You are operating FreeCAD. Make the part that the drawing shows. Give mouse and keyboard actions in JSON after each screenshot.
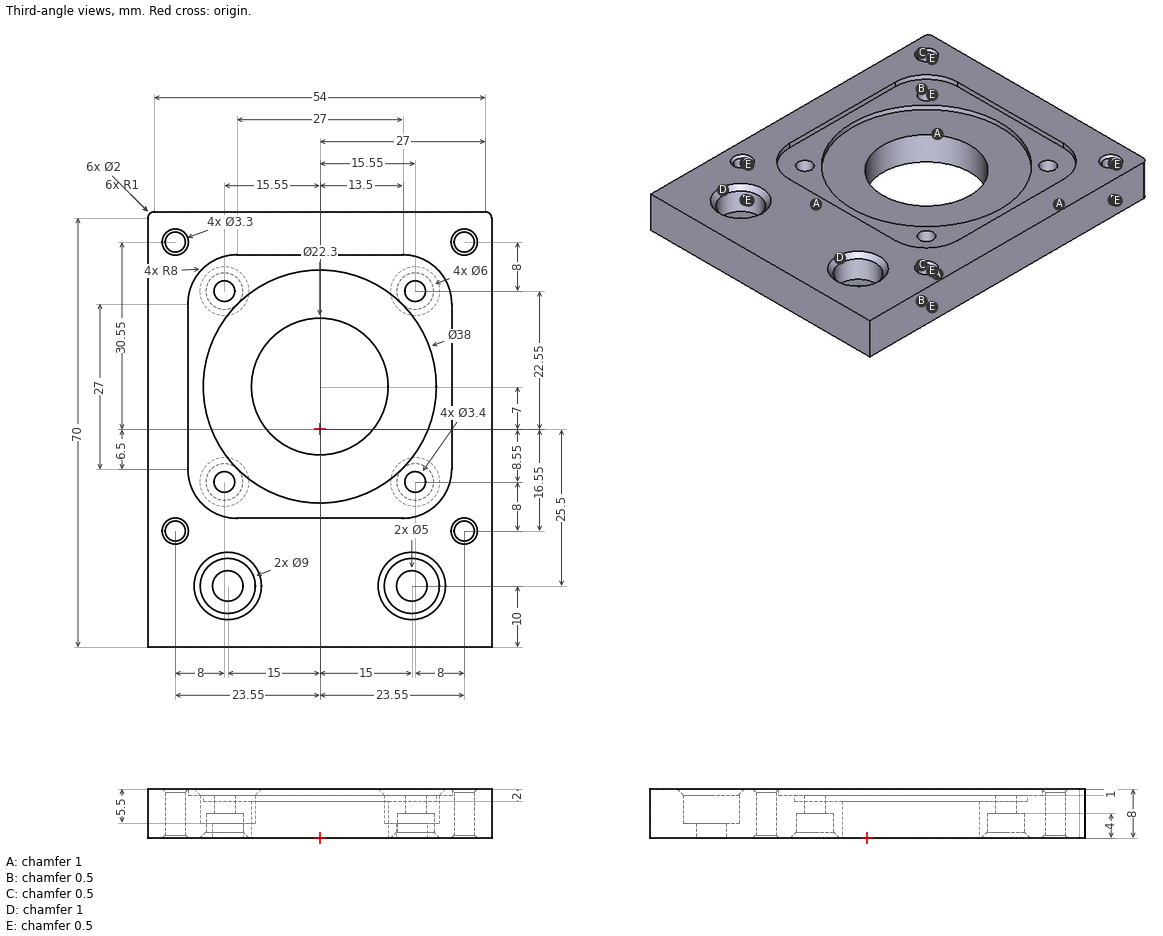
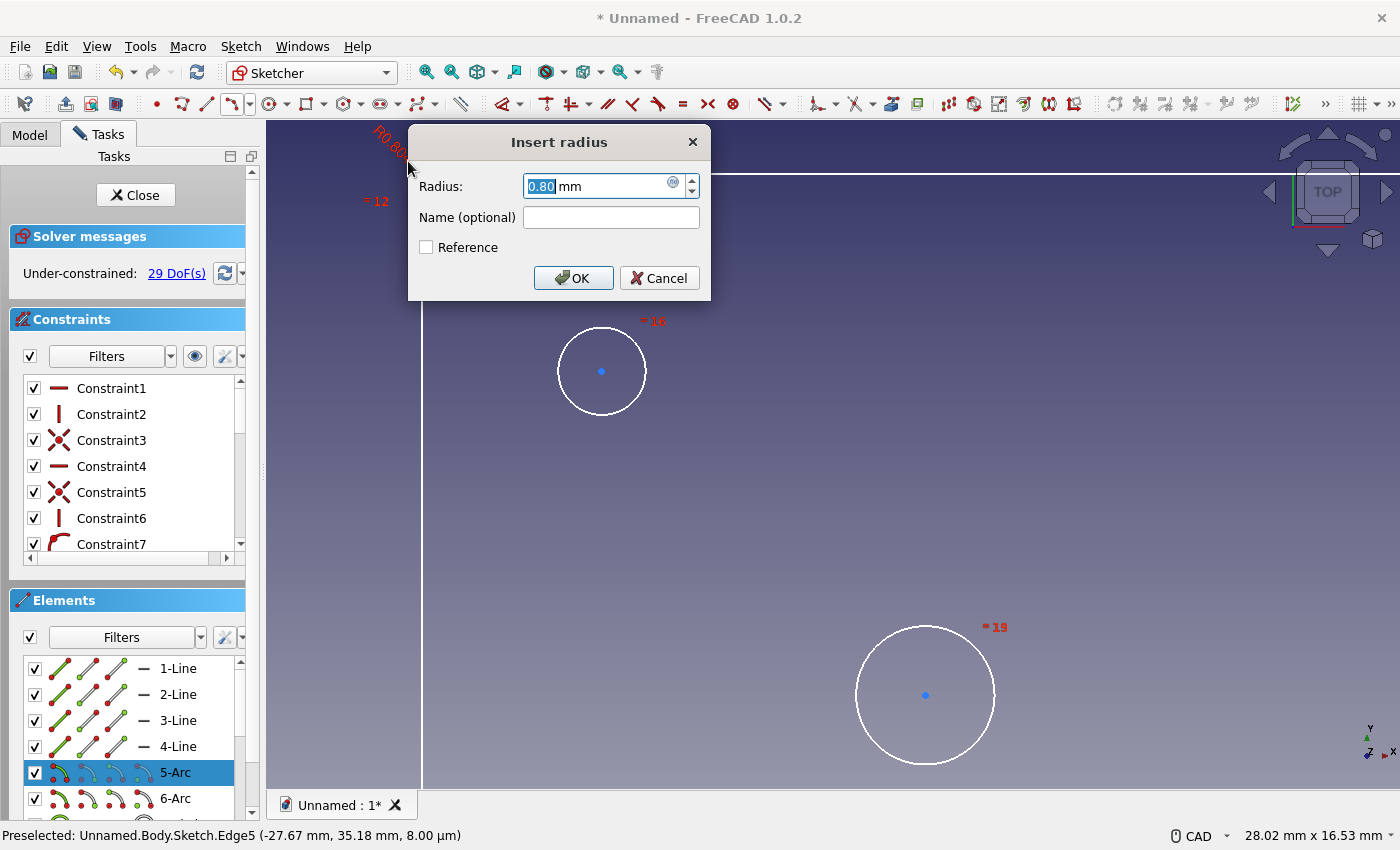
{"action": "type", "text": "1"}
{"action": "key", "text": "Return"}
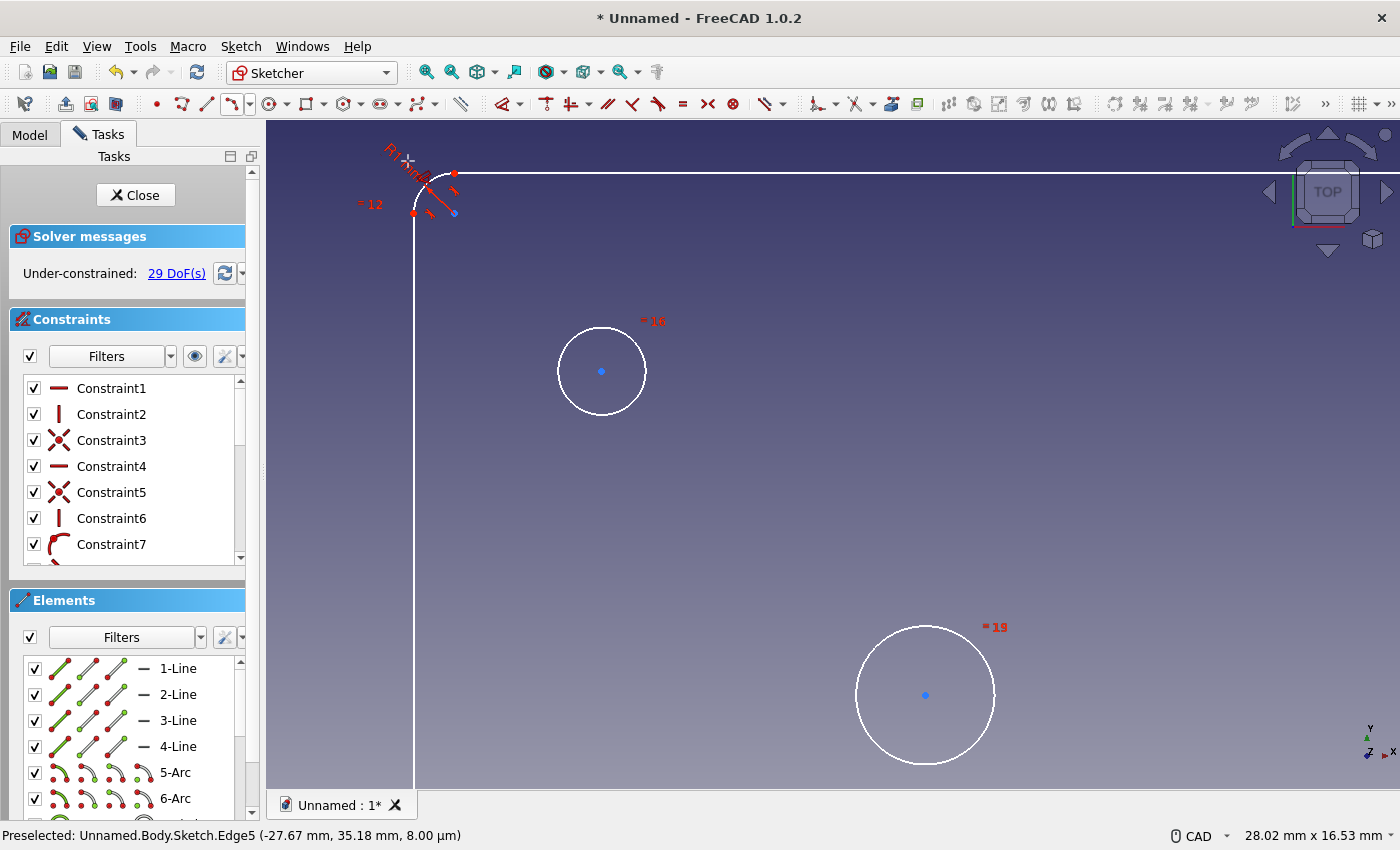
{"action": "scroll", "coordinate": [608, 227], "scroll_direction": "down", "scroll_amount": 9}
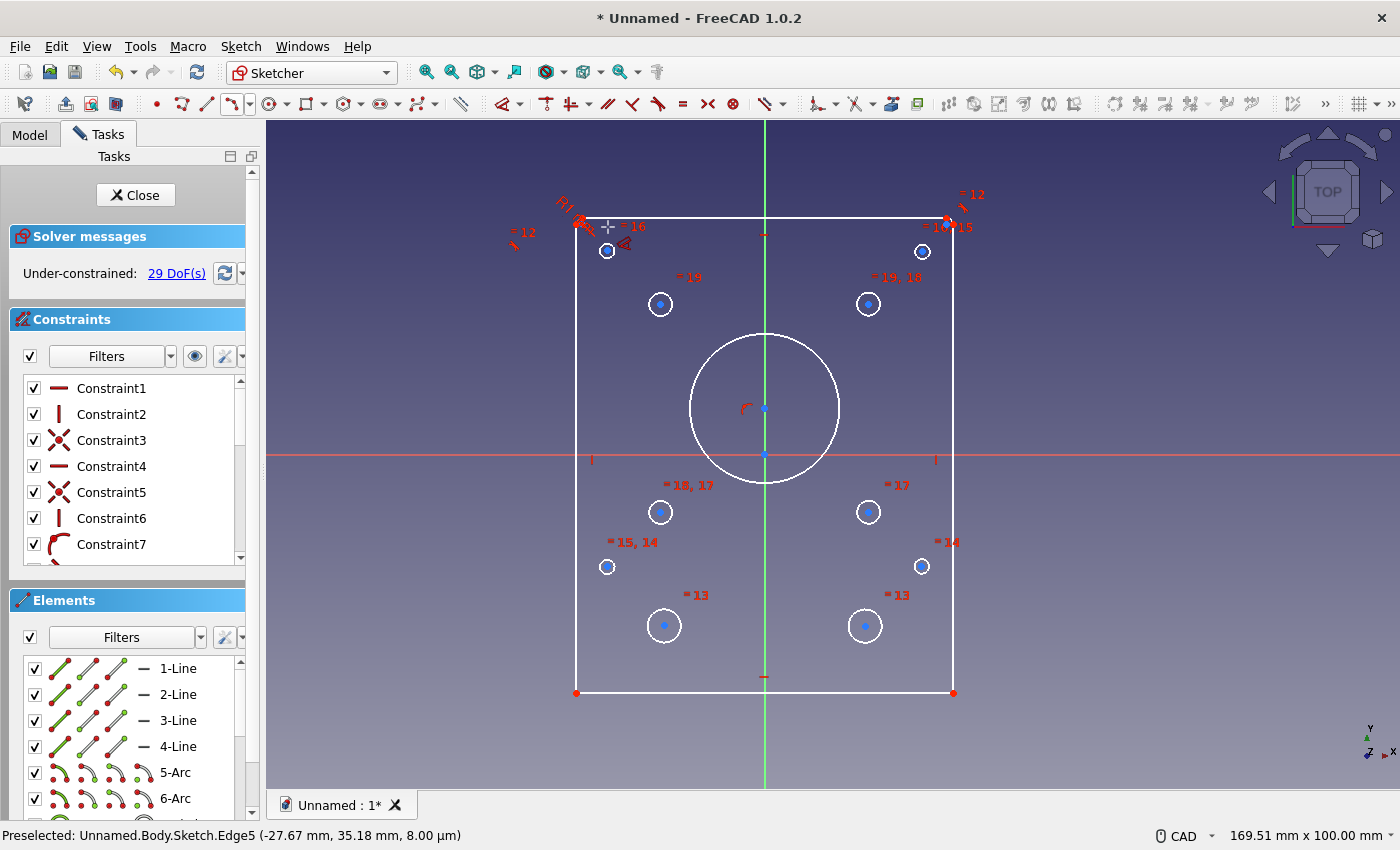
{"action": "left_click", "coordinate": [877, 614]}
{"action": "left_click", "coordinate": [899, 591]}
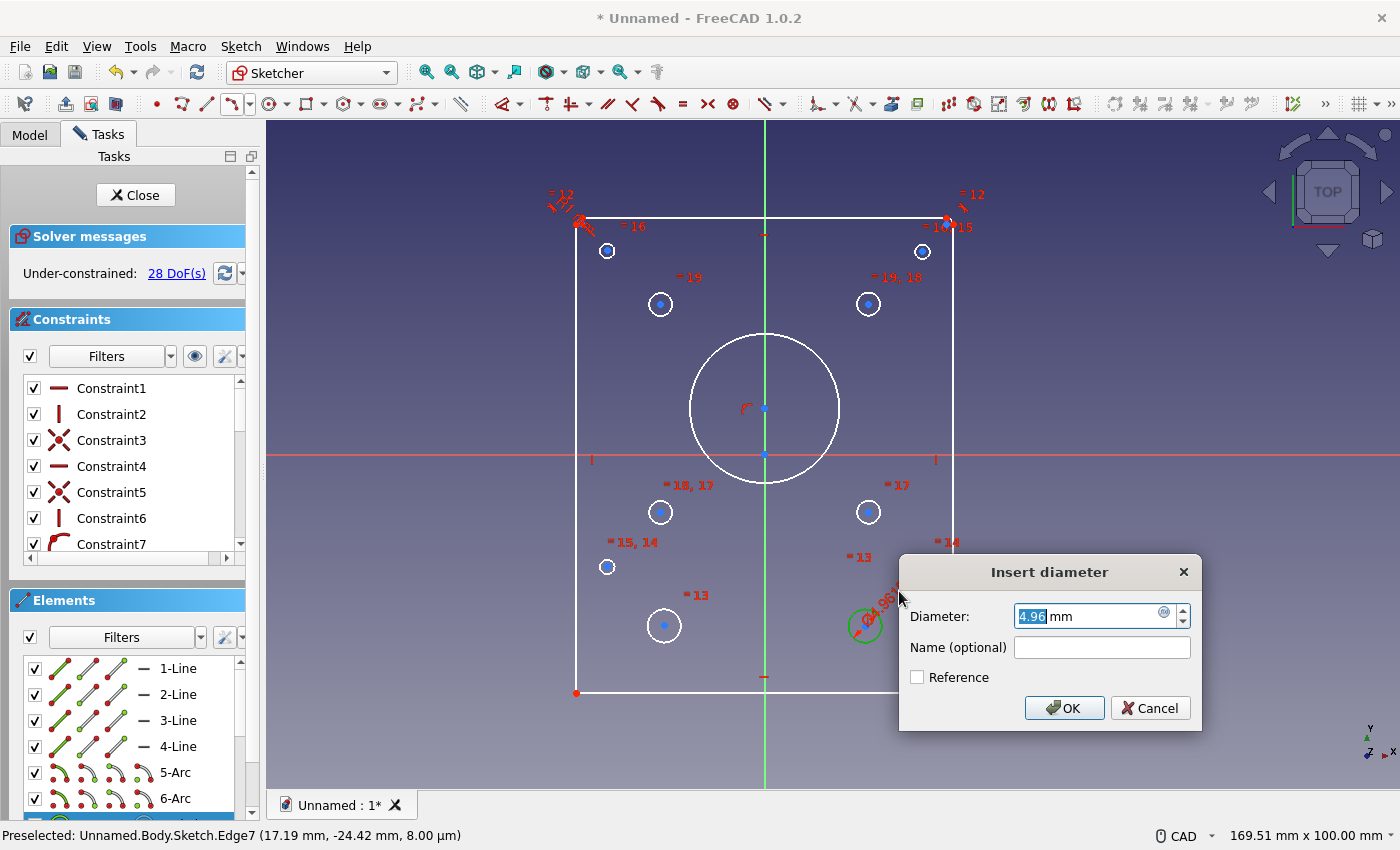
{"action": "type", "text": "5"}
{"action": "key", "text": "Return"}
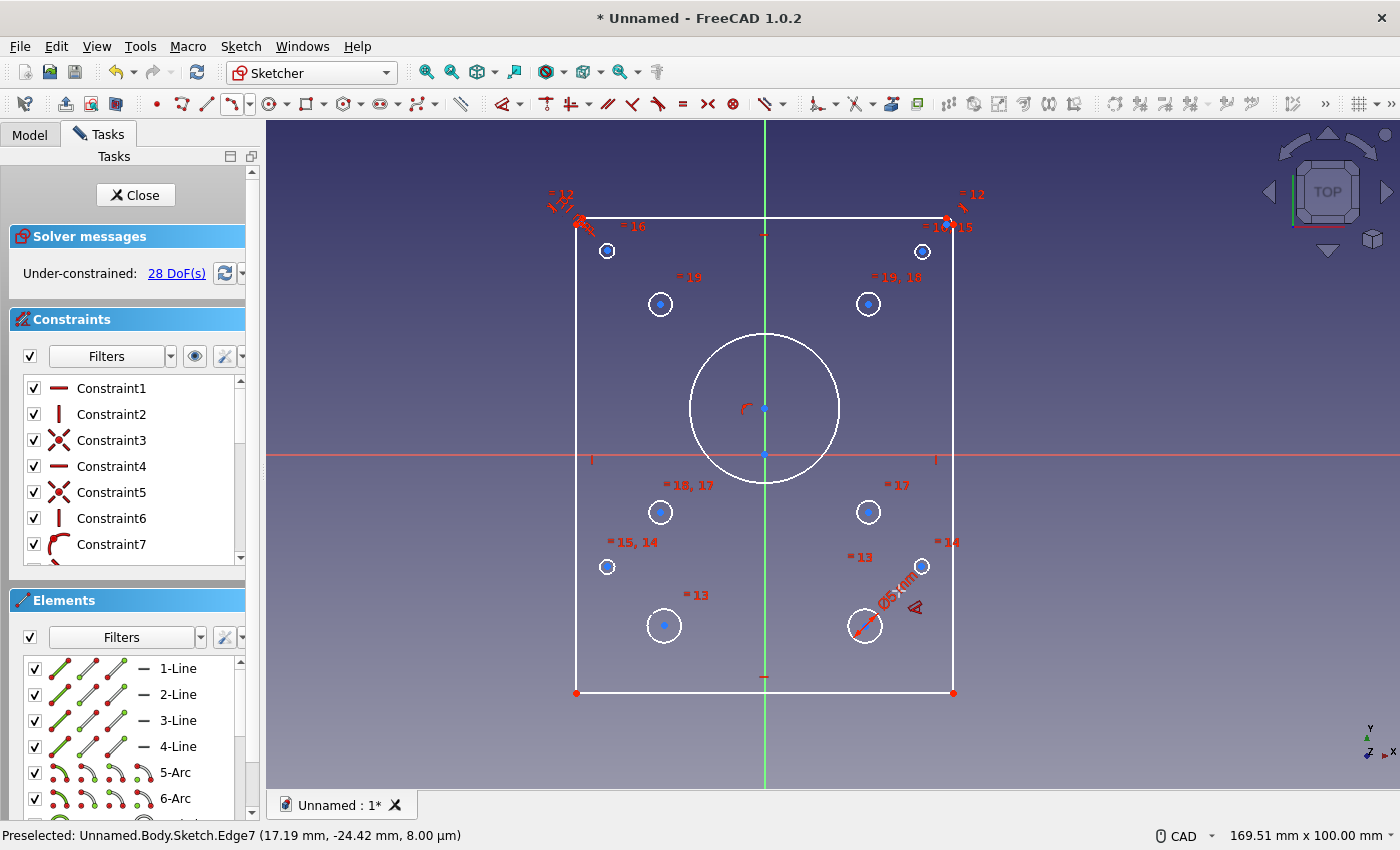
{"action": "scroll", "coordinate": [917, 561], "scroll_direction": "up", "scroll_amount": 6}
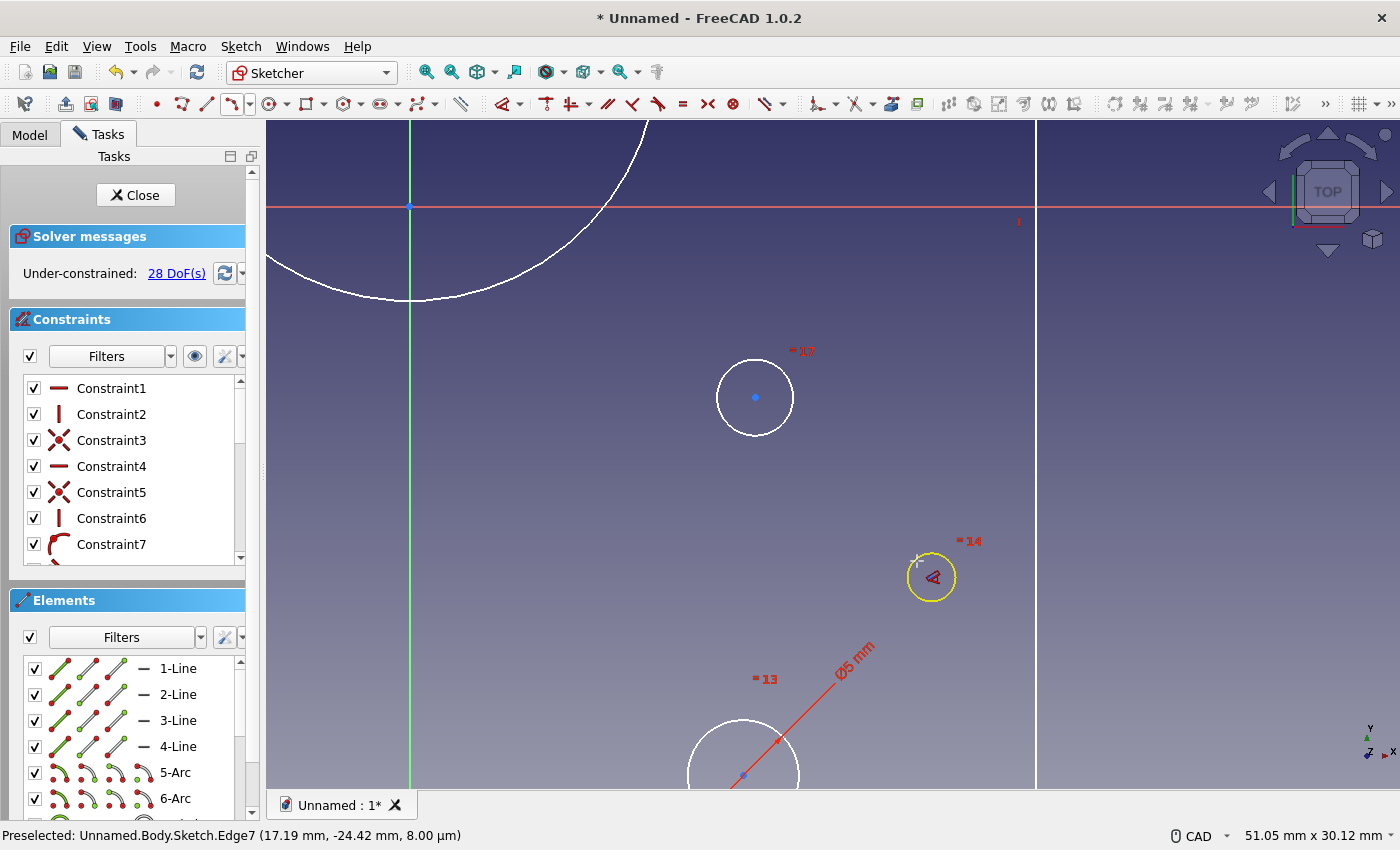
{"action": "left_click", "coordinate": [915, 560]}
{"action": "left_click", "coordinate": [893, 537]}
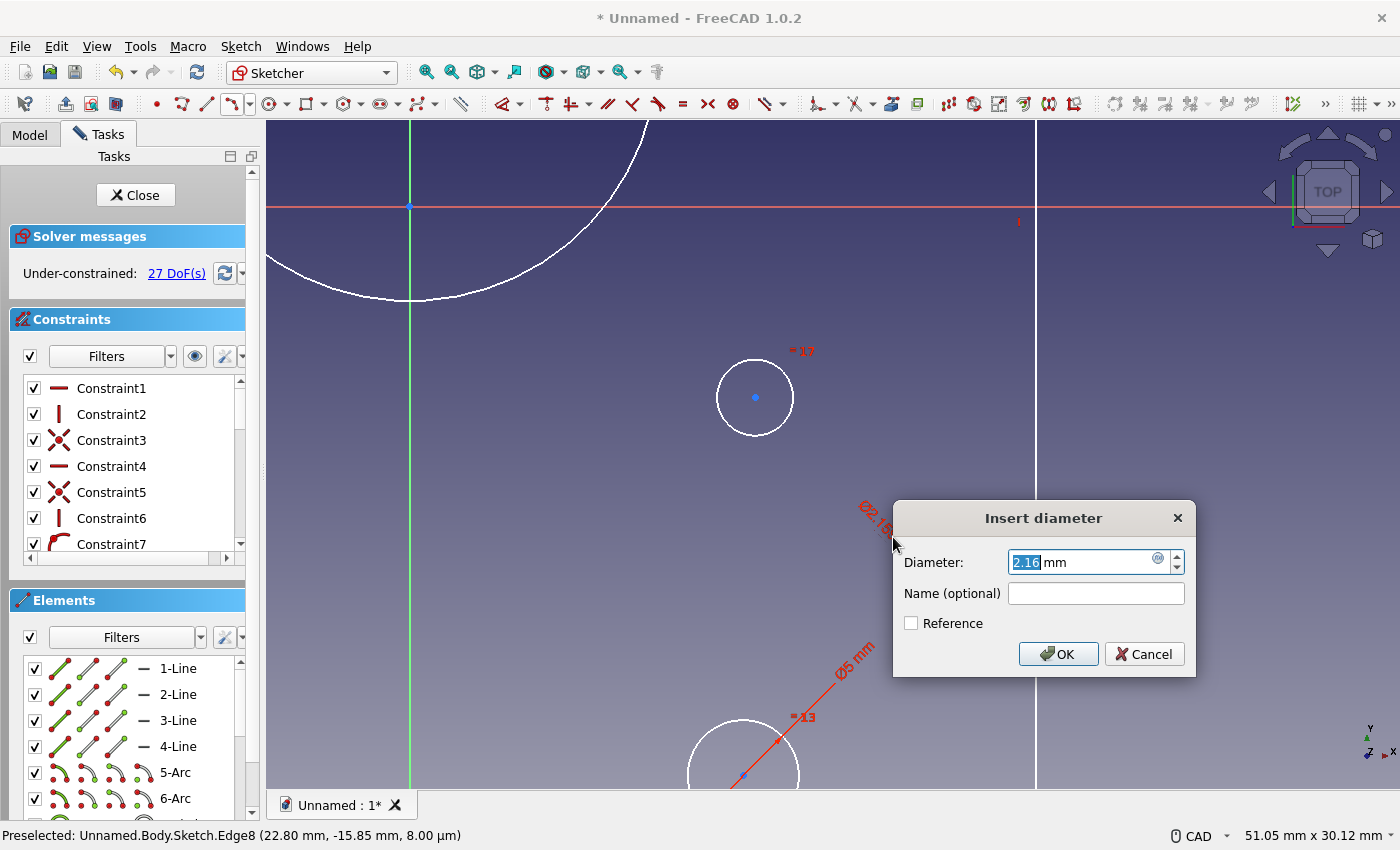
{"action": "type", "text": "2"}
{"action": "key", "text": "Return"}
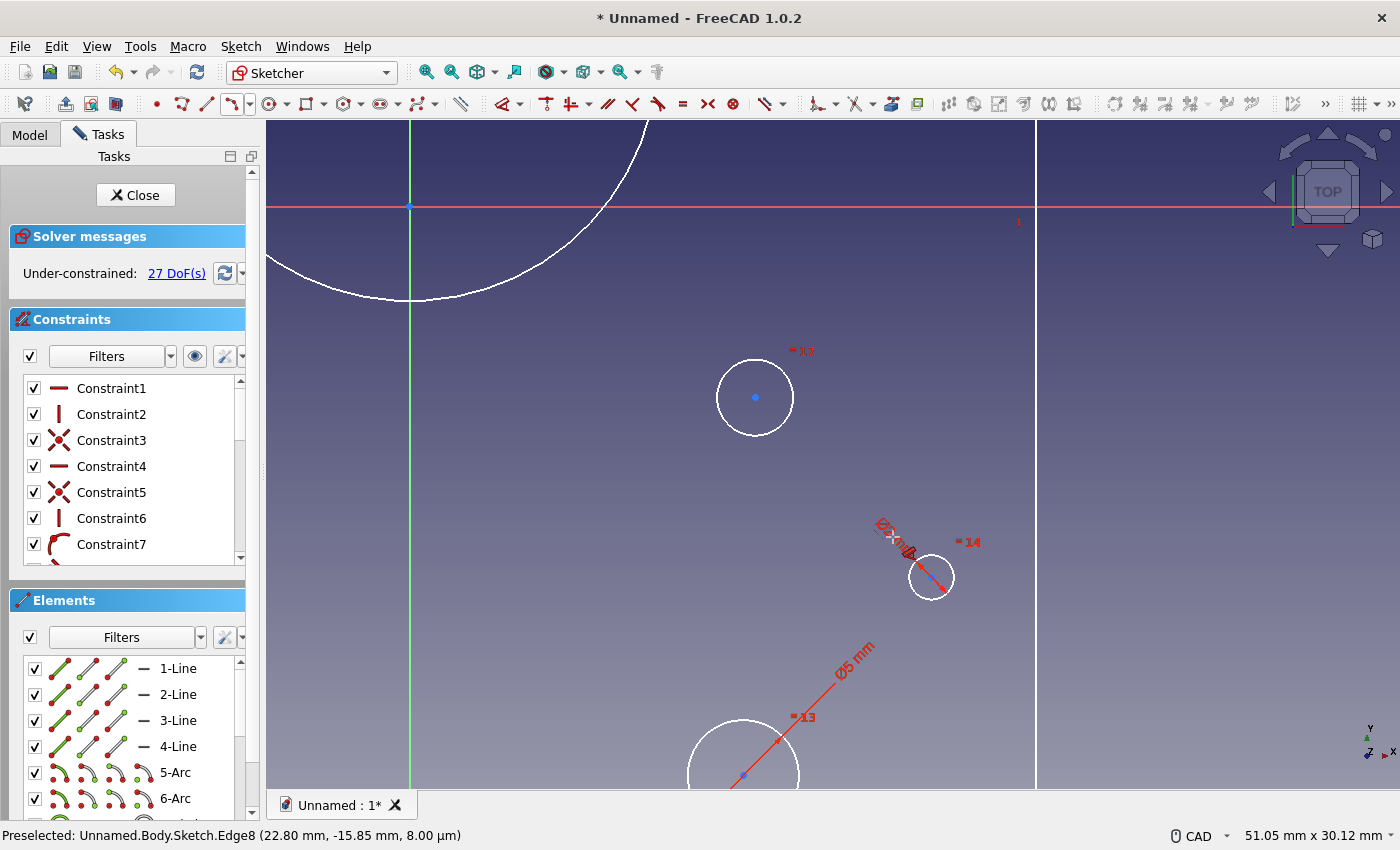
{"action": "left_click", "coordinate": [782, 371]}
{"action": "left_click", "coordinate": [805, 348]}